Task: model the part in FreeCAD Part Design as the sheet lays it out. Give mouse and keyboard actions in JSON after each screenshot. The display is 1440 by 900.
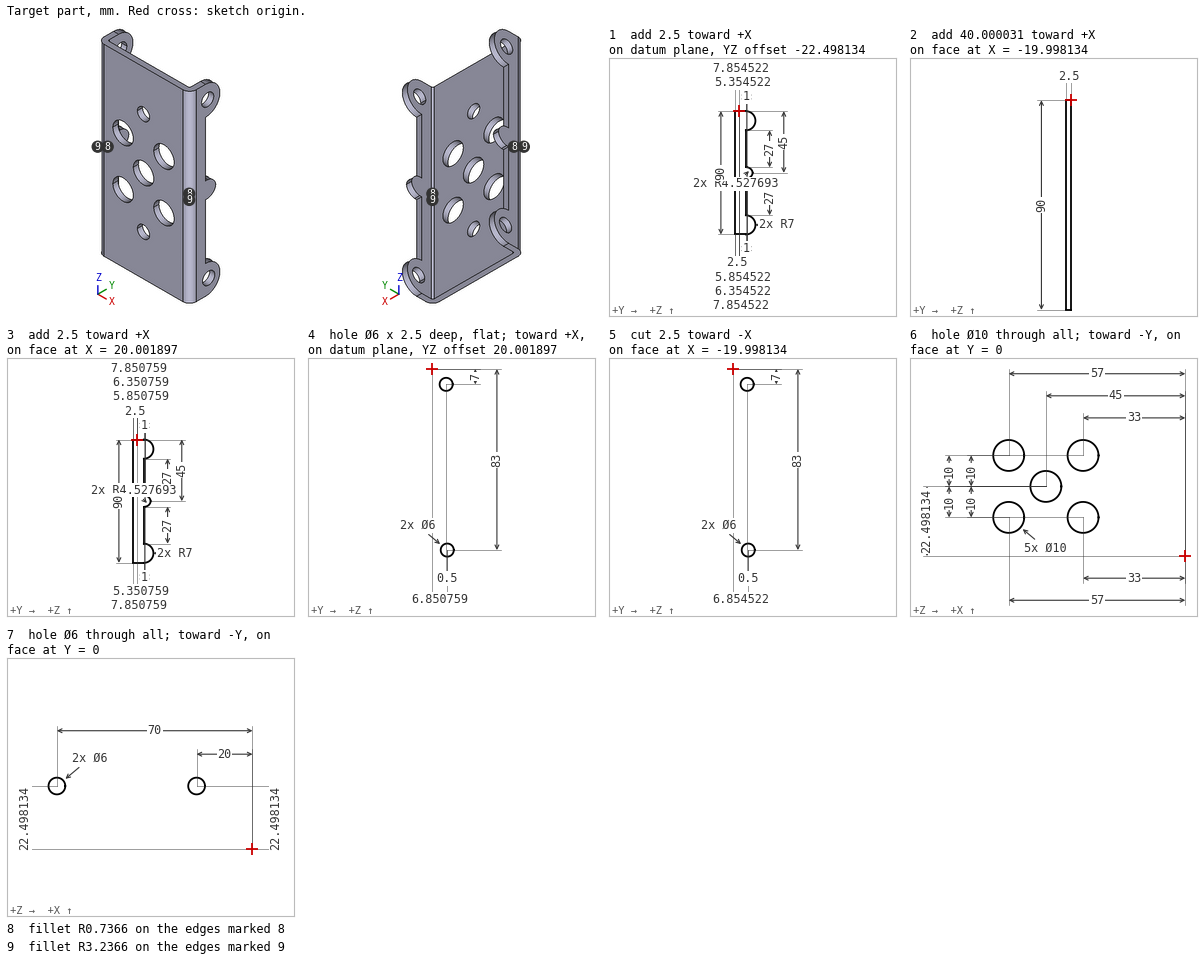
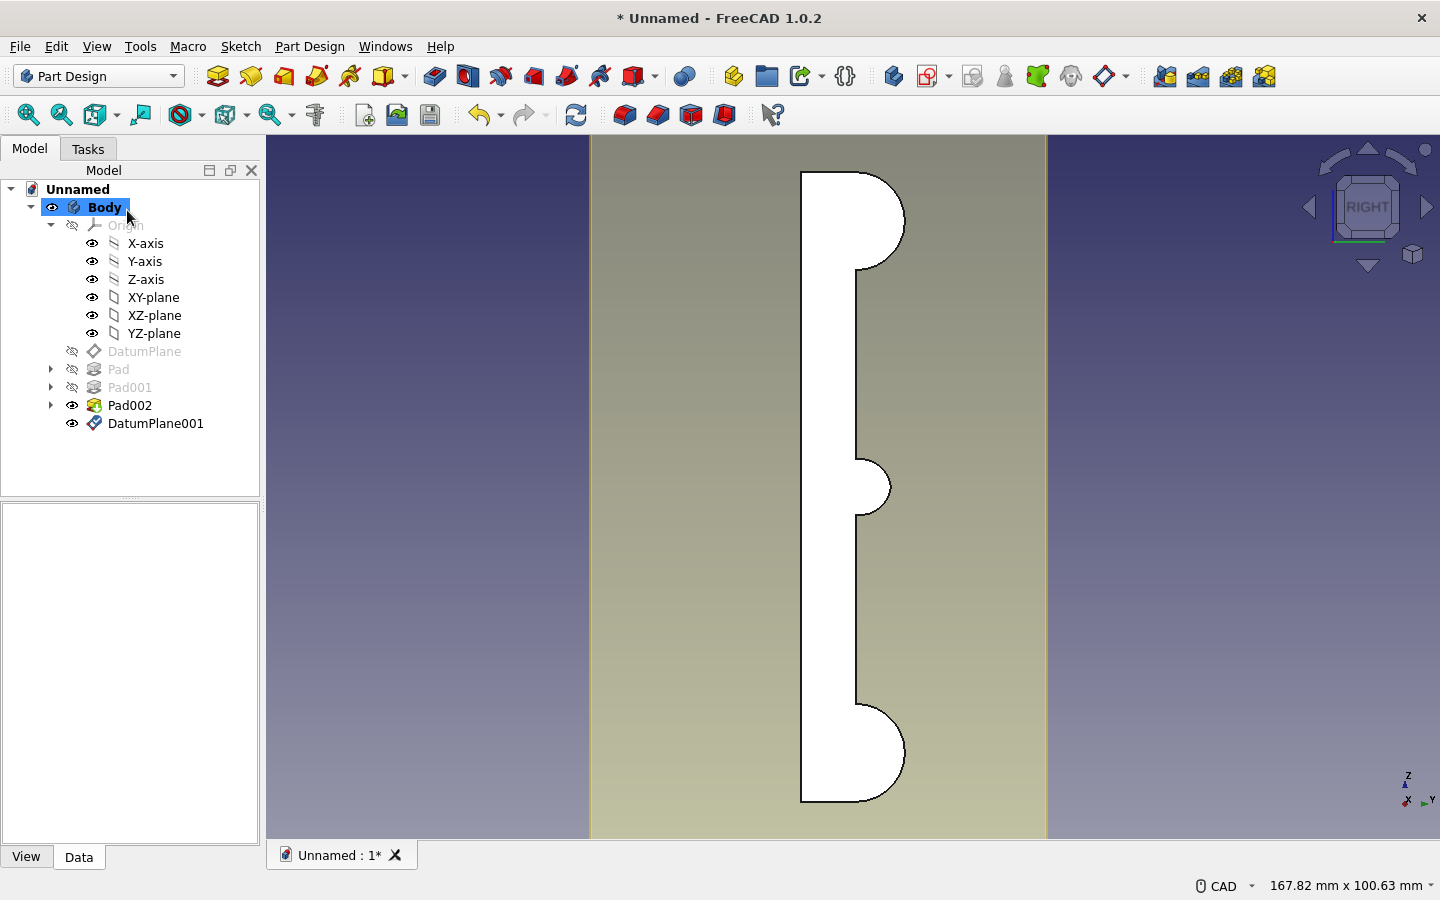
{"action": "left_click", "coordinate": [117, 423]}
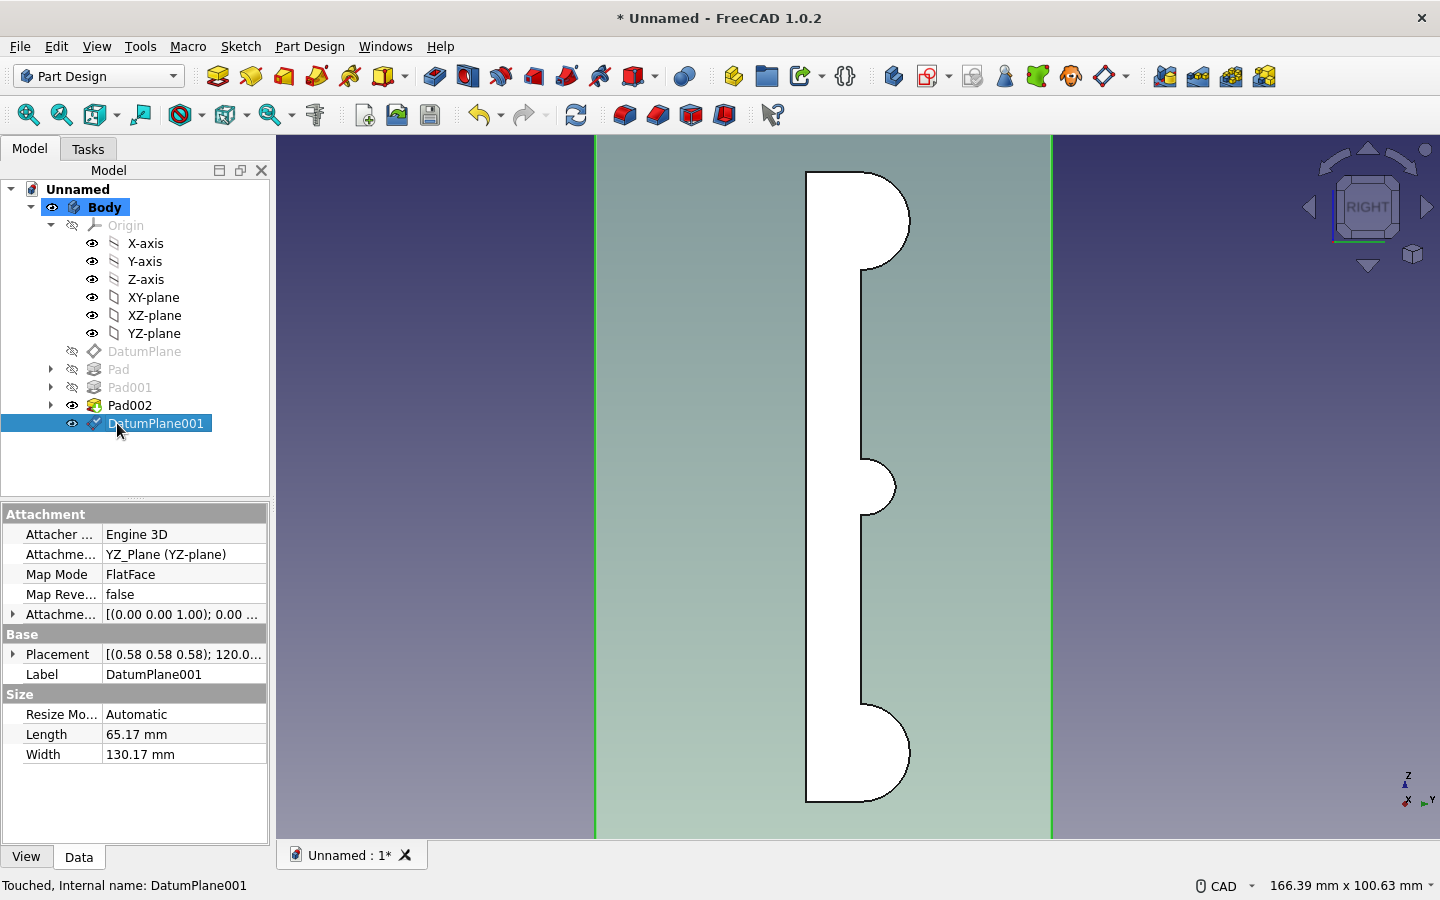
{"action": "left_click", "coordinate": [926, 76]}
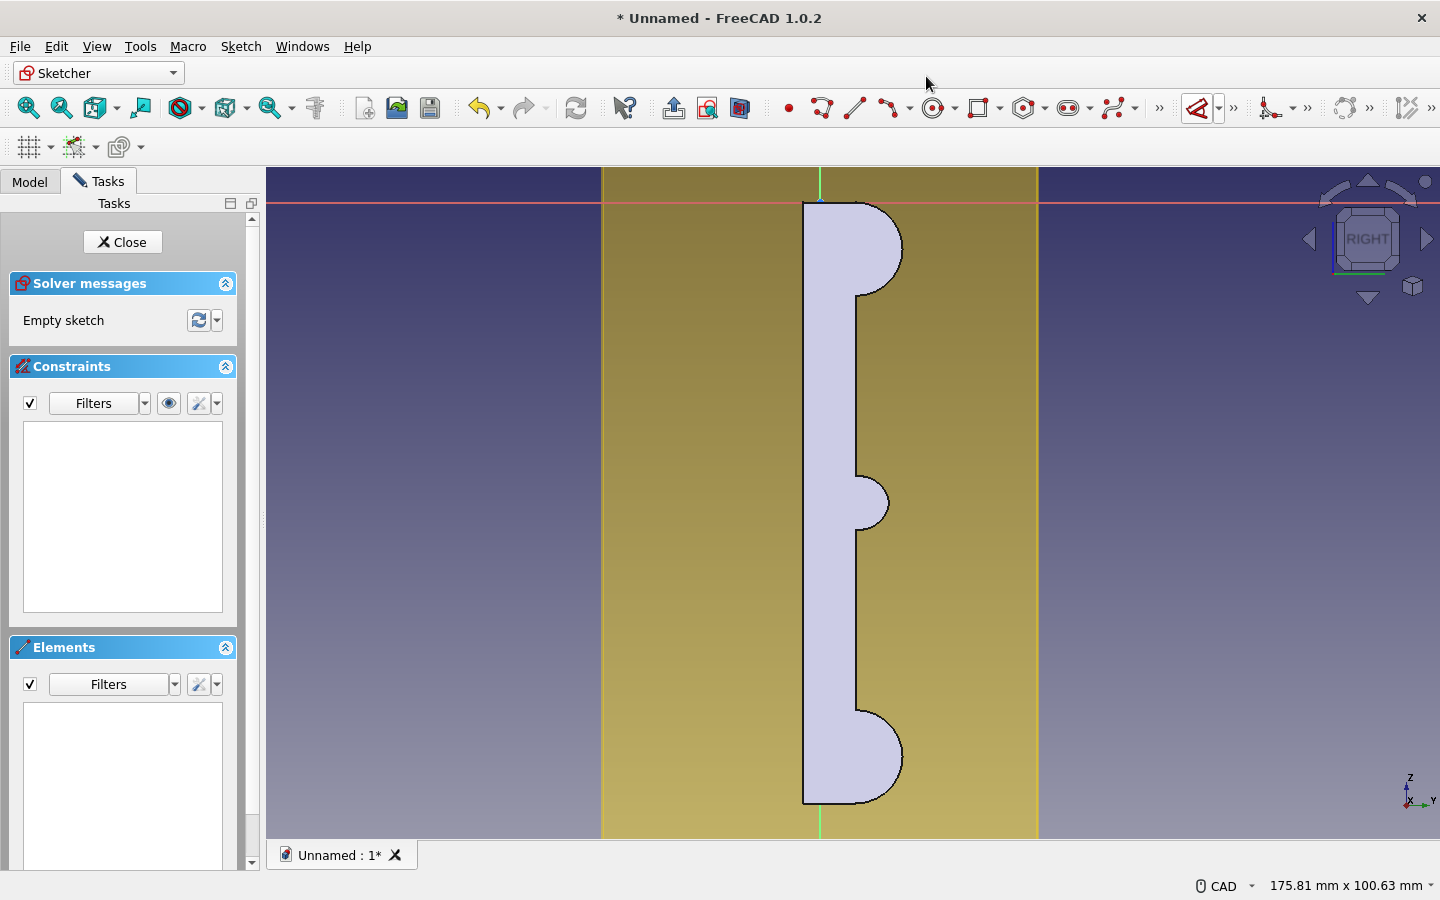
{"action": "left_click", "coordinate": [740, 108]}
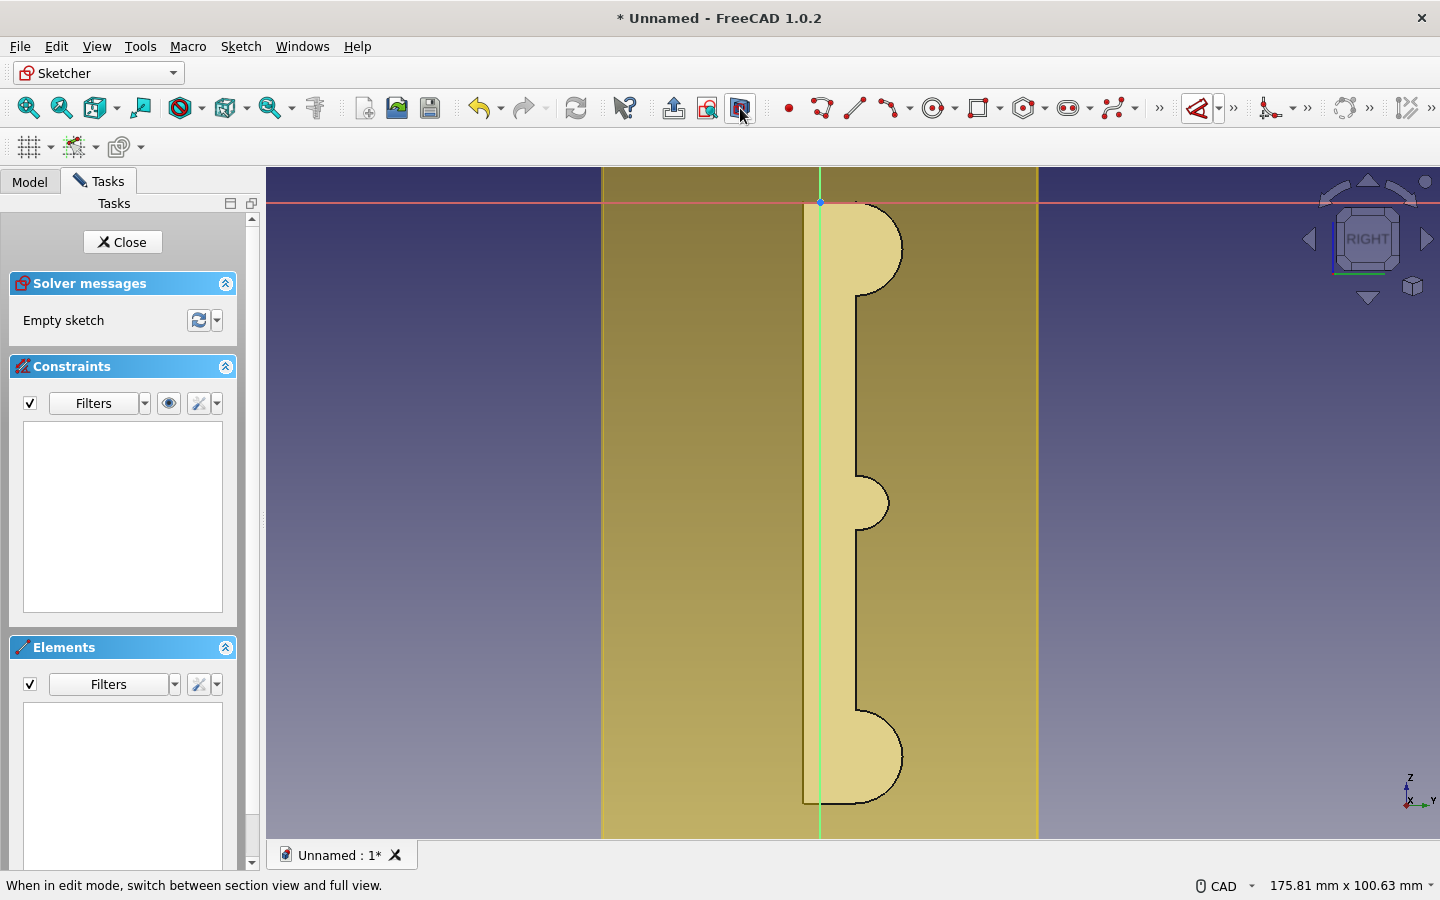
{"action": "scroll", "coordinate": [475, 563], "scroll_direction": "down", "scroll_amount": 1}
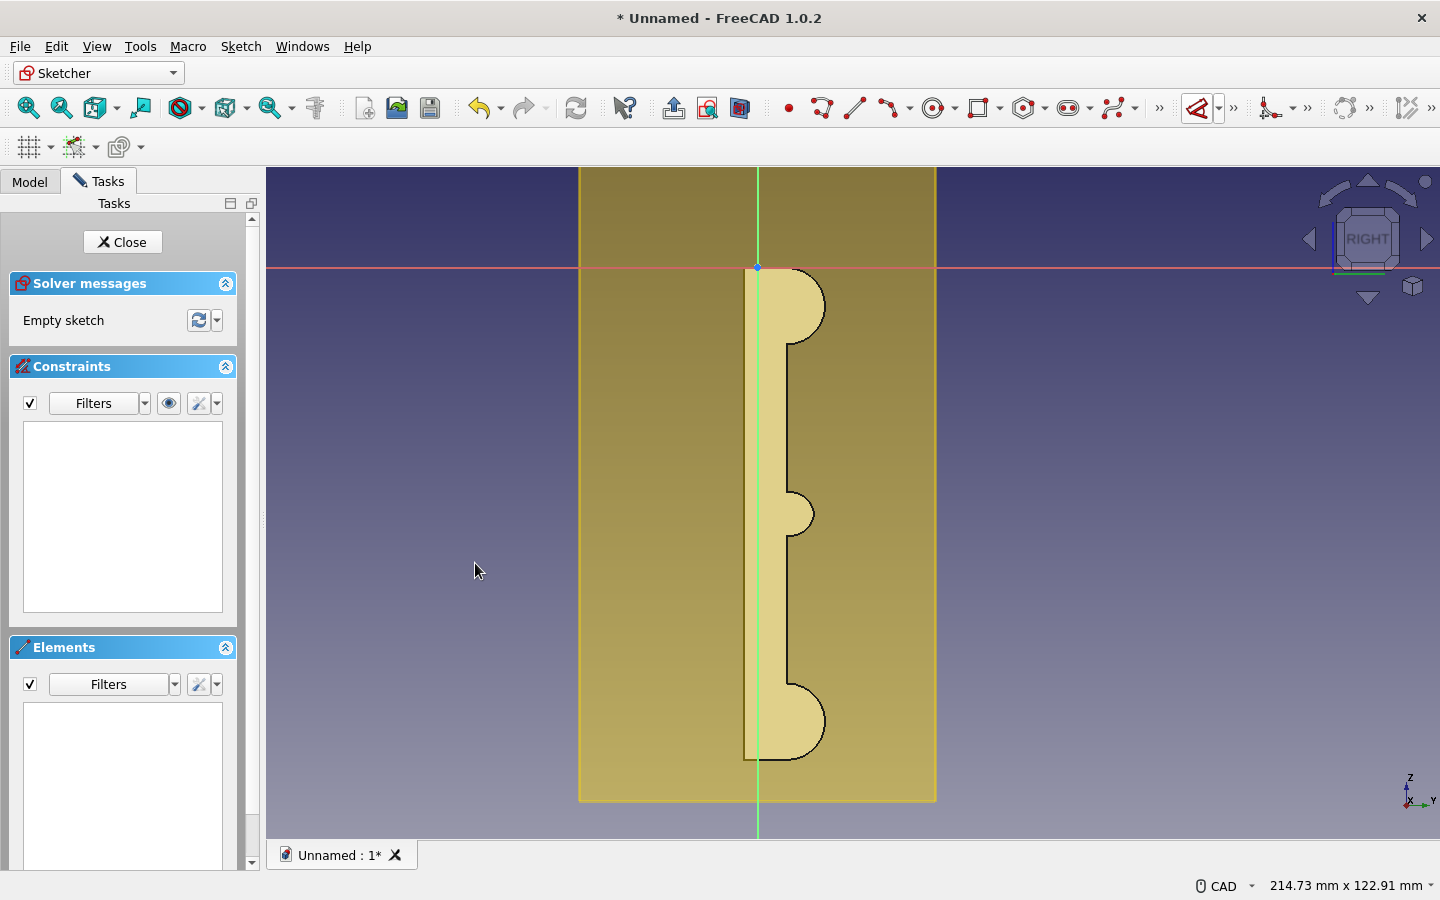
{"action": "key", "text": "g c"}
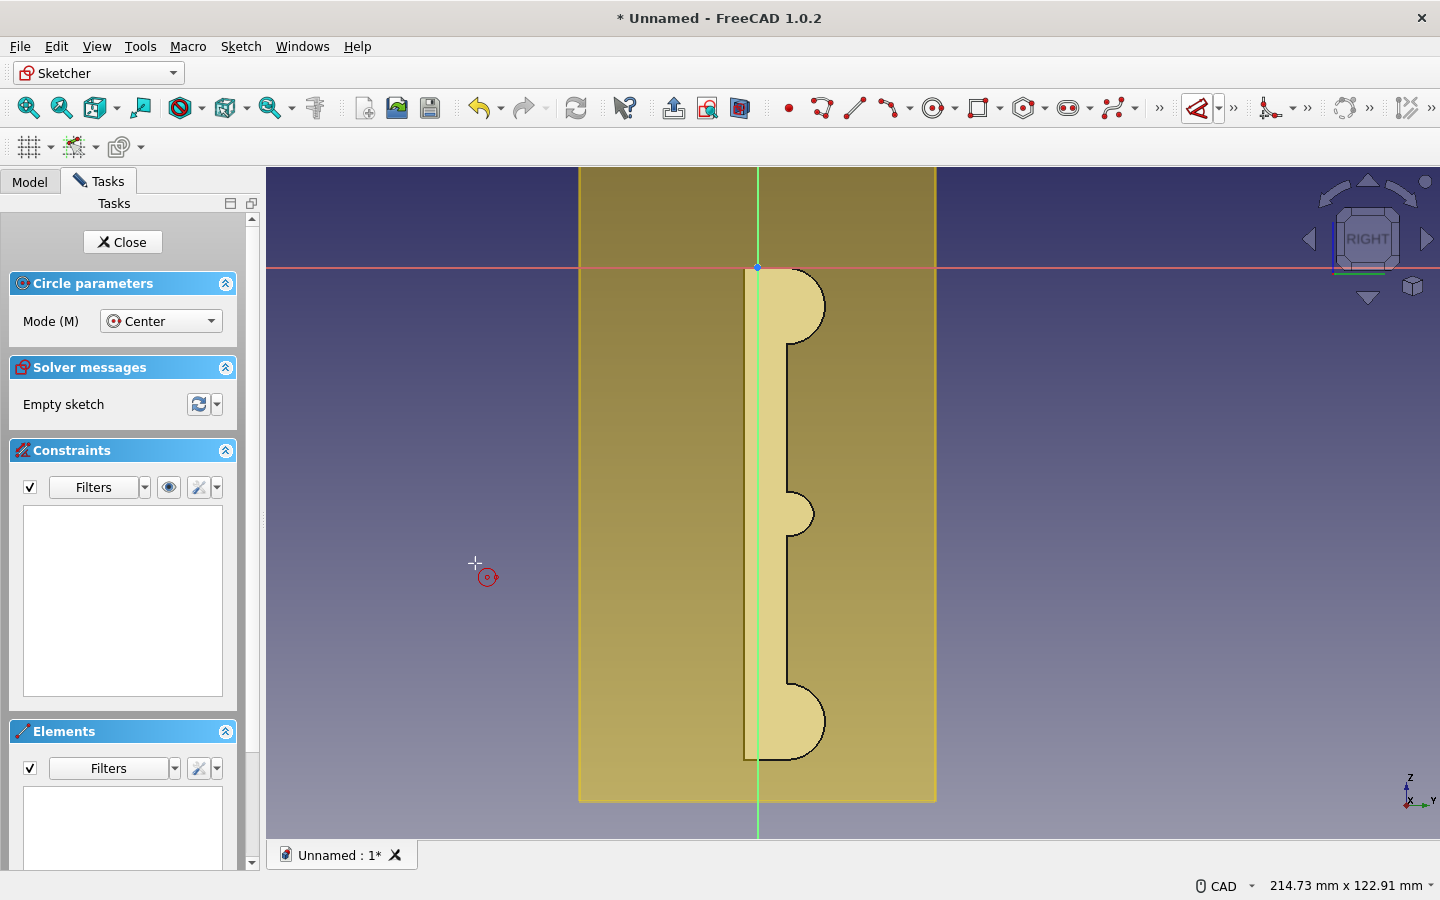
{"action": "scroll", "coordinate": [795, 722], "scroll_direction": "up", "scroll_amount": 2}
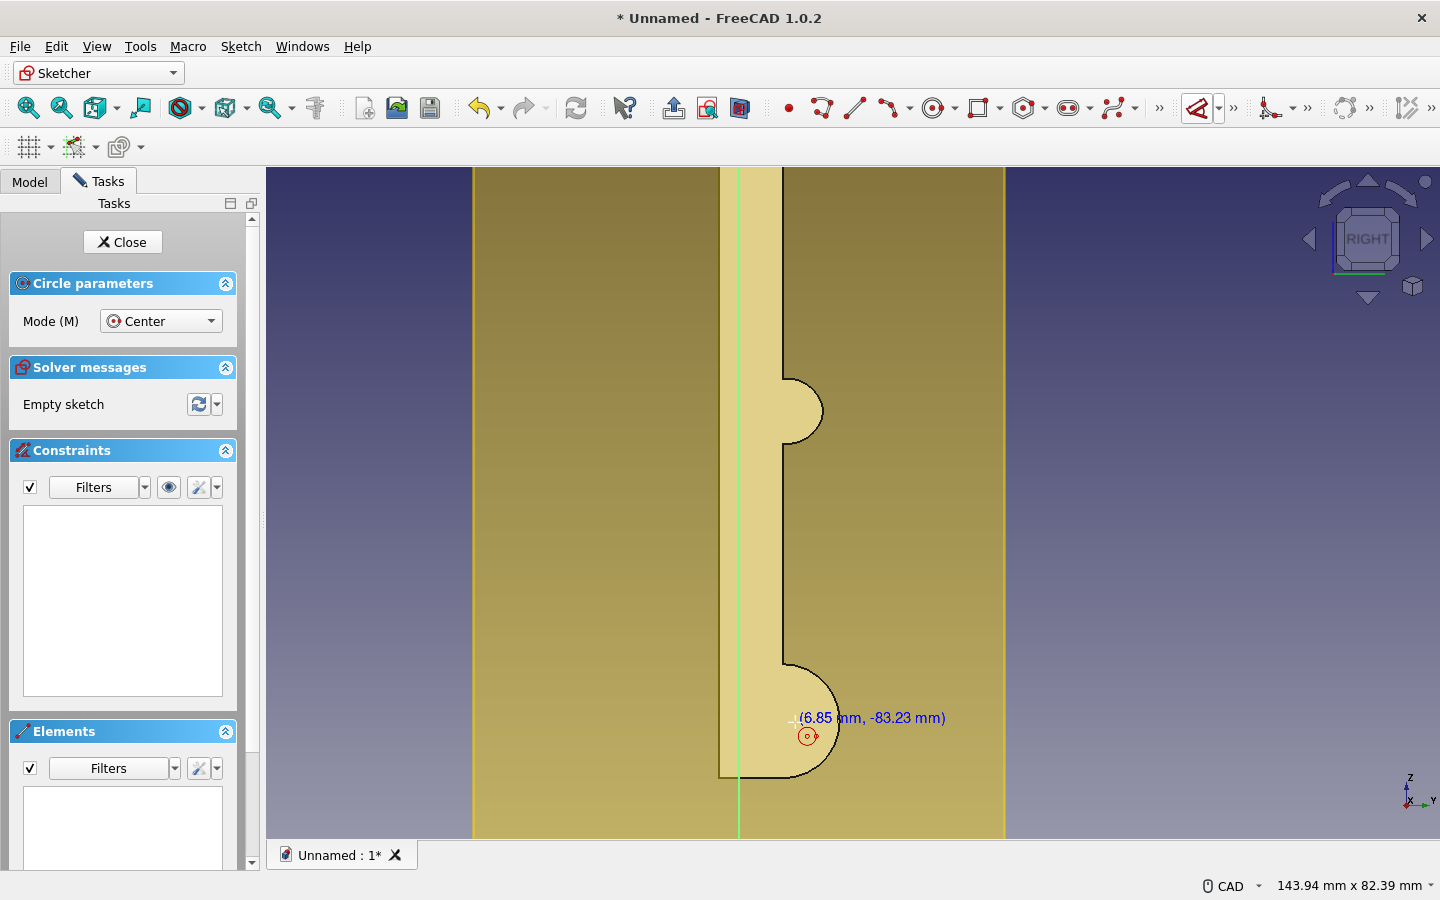
{"action": "left_click", "coordinate": [795, 721]}
{"action": "mouse_move", "coordinate": [812, 704]}